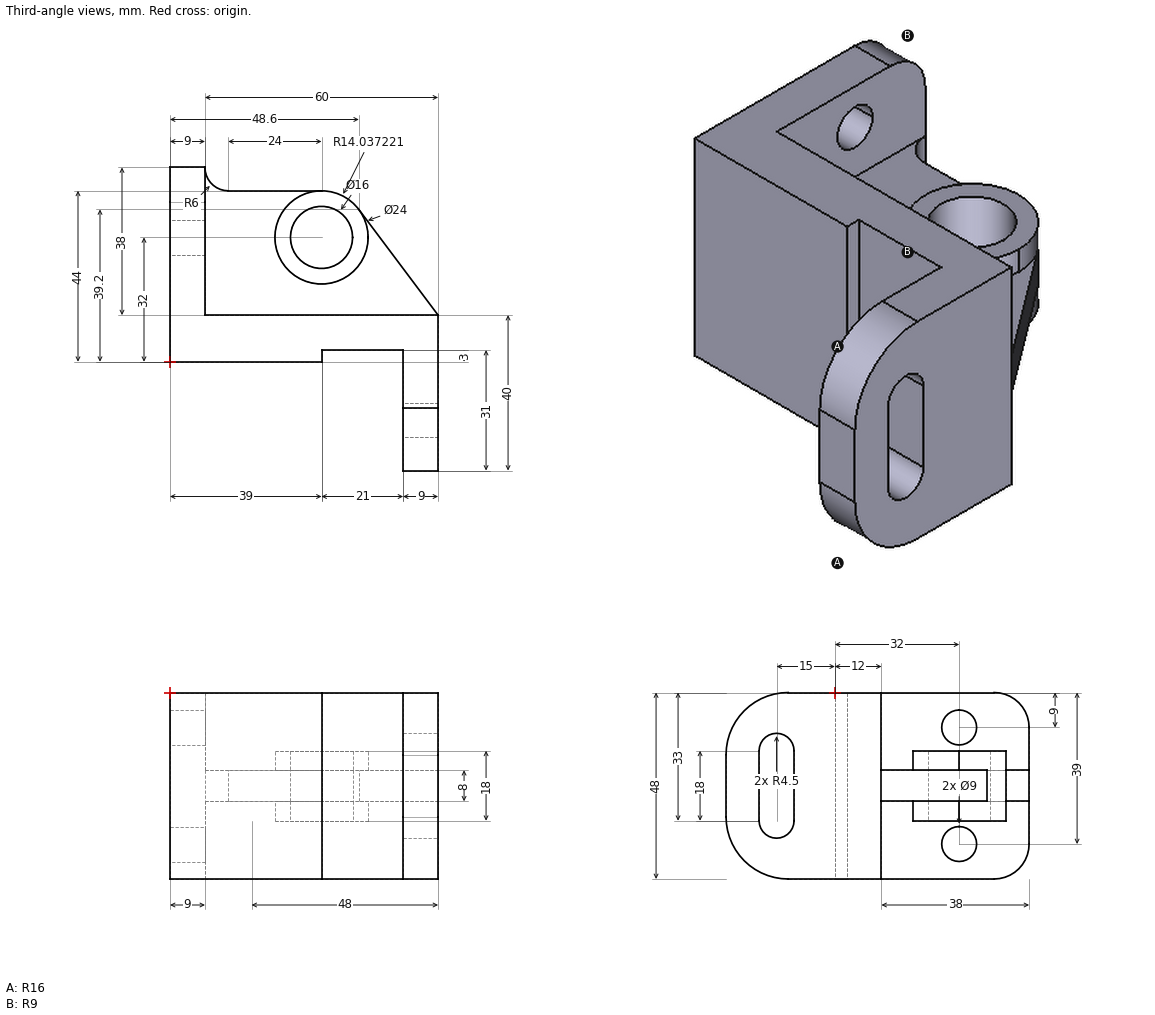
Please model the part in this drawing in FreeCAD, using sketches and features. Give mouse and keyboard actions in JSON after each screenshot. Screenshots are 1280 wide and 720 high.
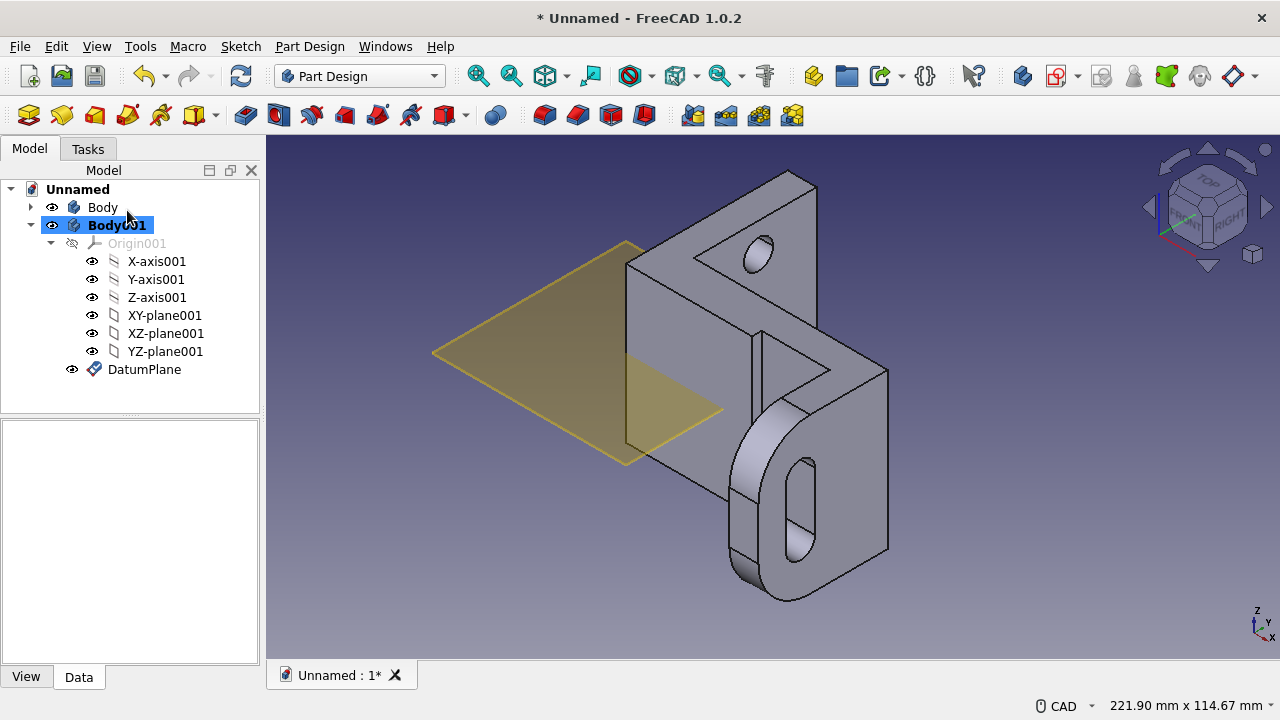
{"action": "left_click", "coordinate": [117, 369]}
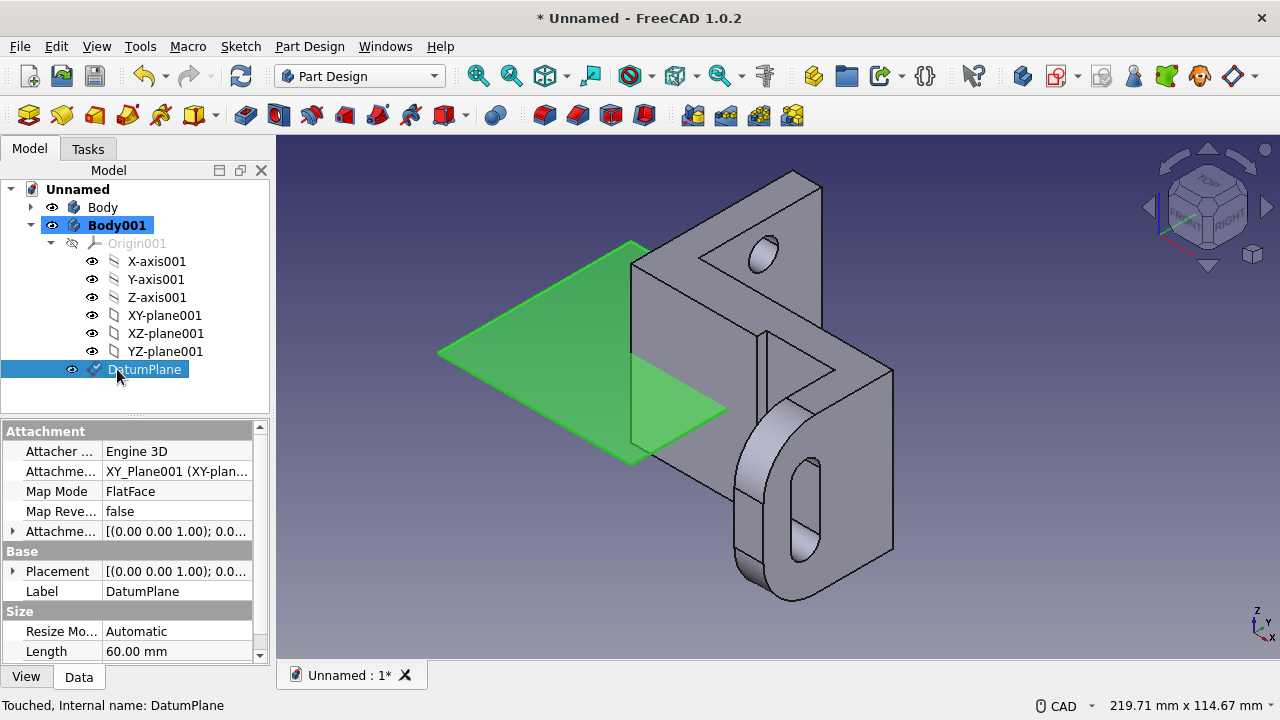
{"action": "left_click", "coordinate": [1056, 76]}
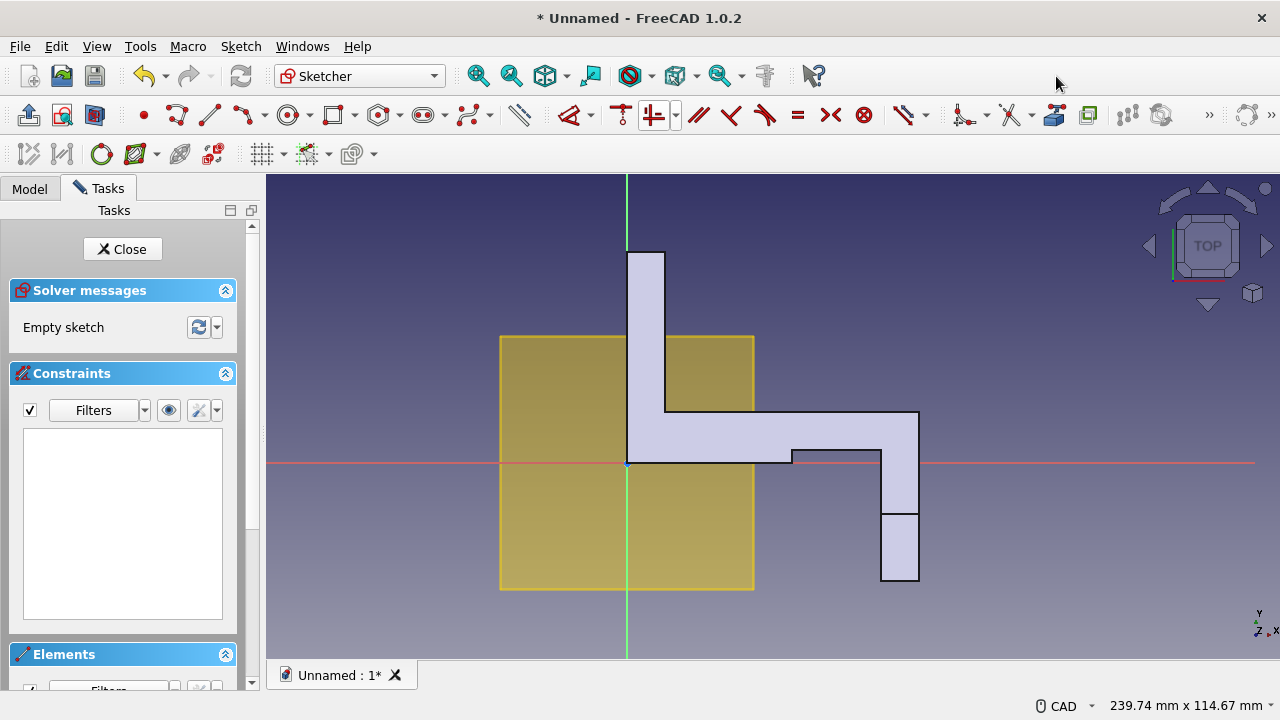
{"action": "scroll", "coordinate": [797, 275], "scroll_direction": "up", "scroll_amount": 2}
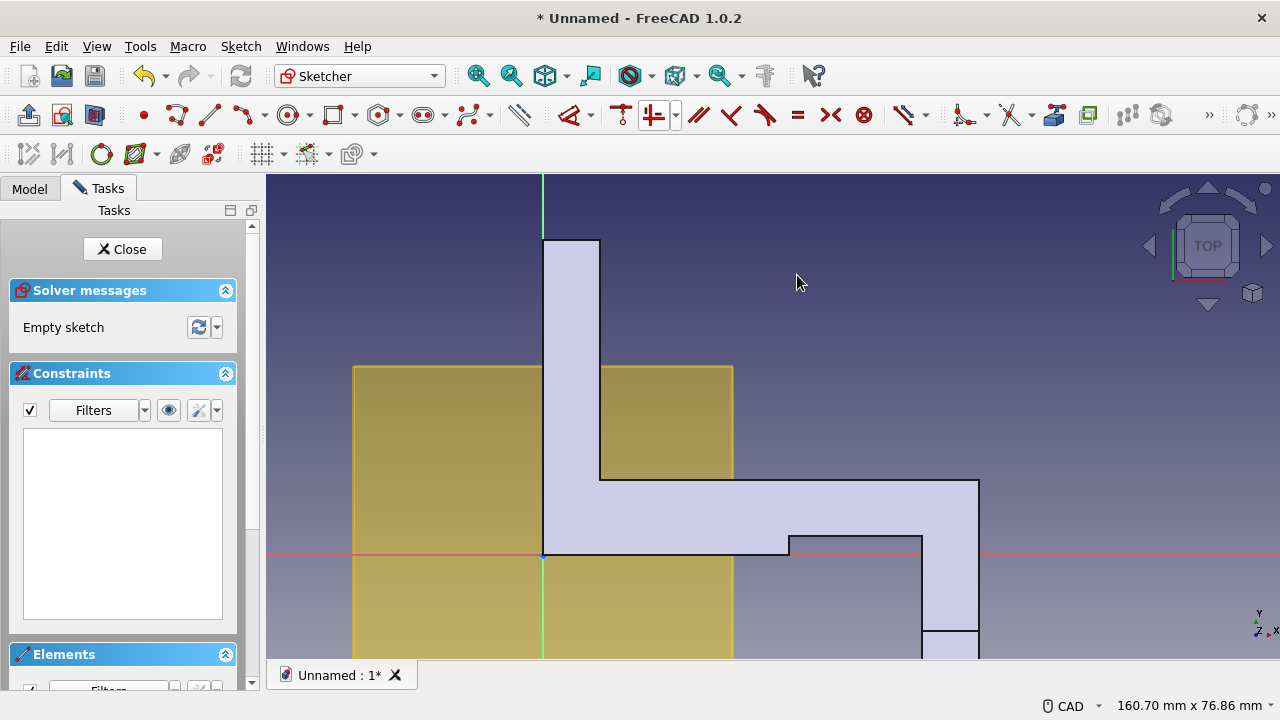
{"action": "key", "text": "g c"}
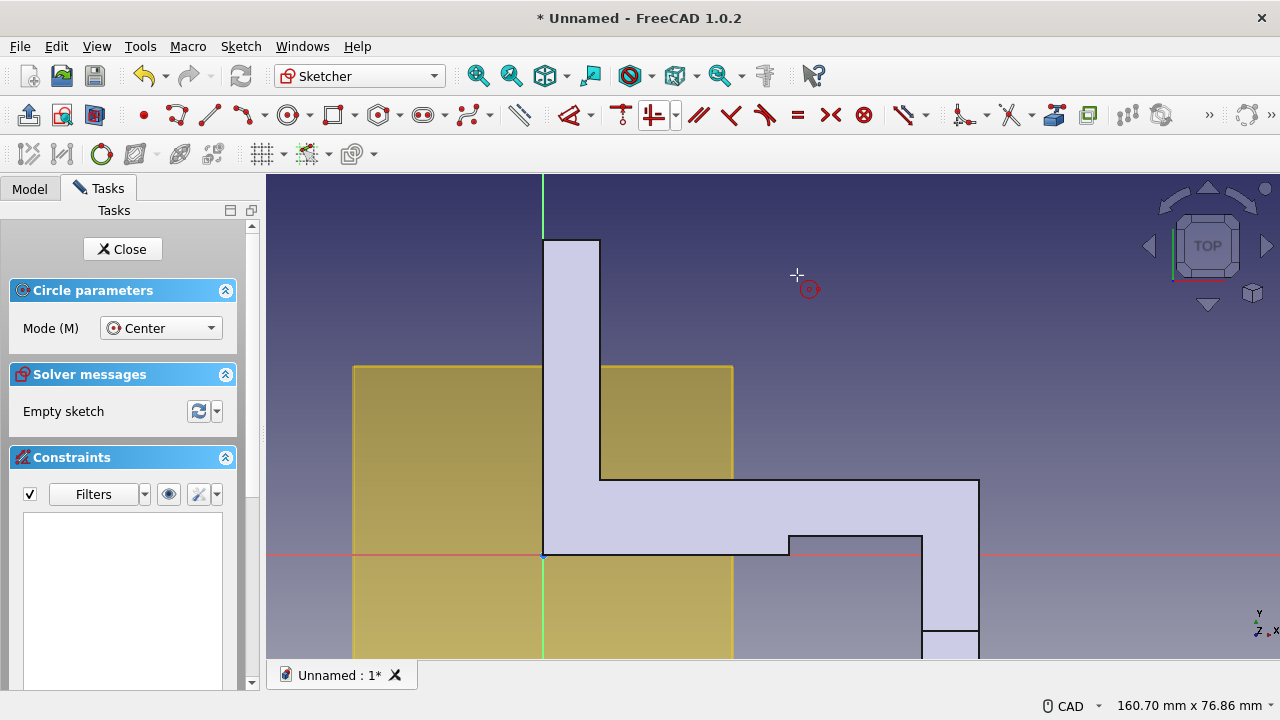
{"action": "left_click", "coordinate": [789, 353]}
{"action": "left_click", "coordinate": [843, 300]}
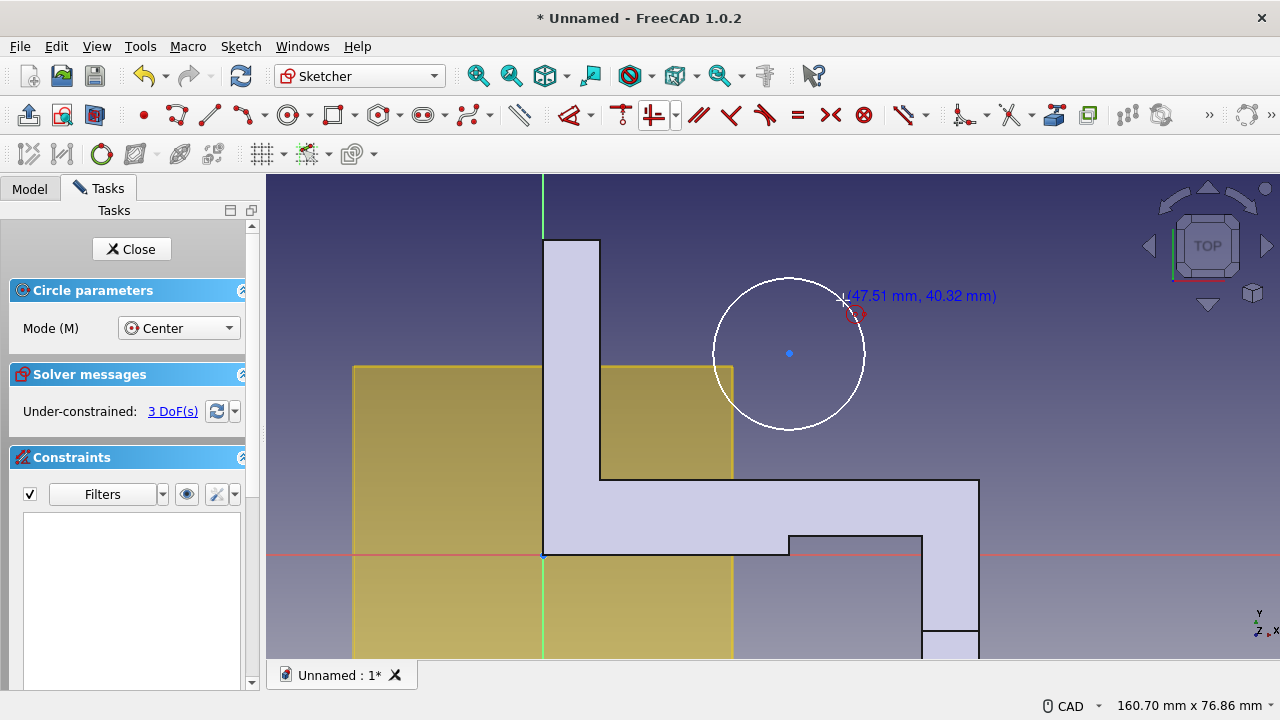
{"action": "left_click", "coordinate": [789, 354]}
{"action": "left_click", "coordinate": [825, 318]}
{"action": "key", "text": "Escape"}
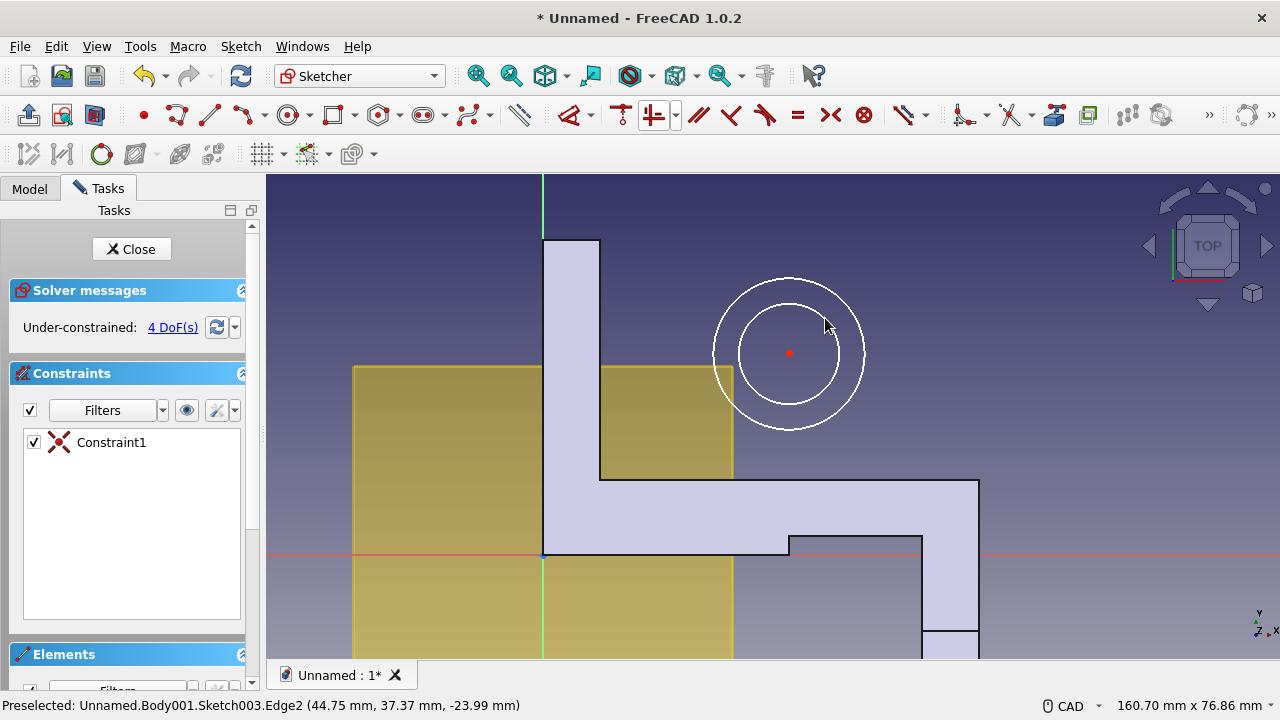
{"action": "key", "text": "d"}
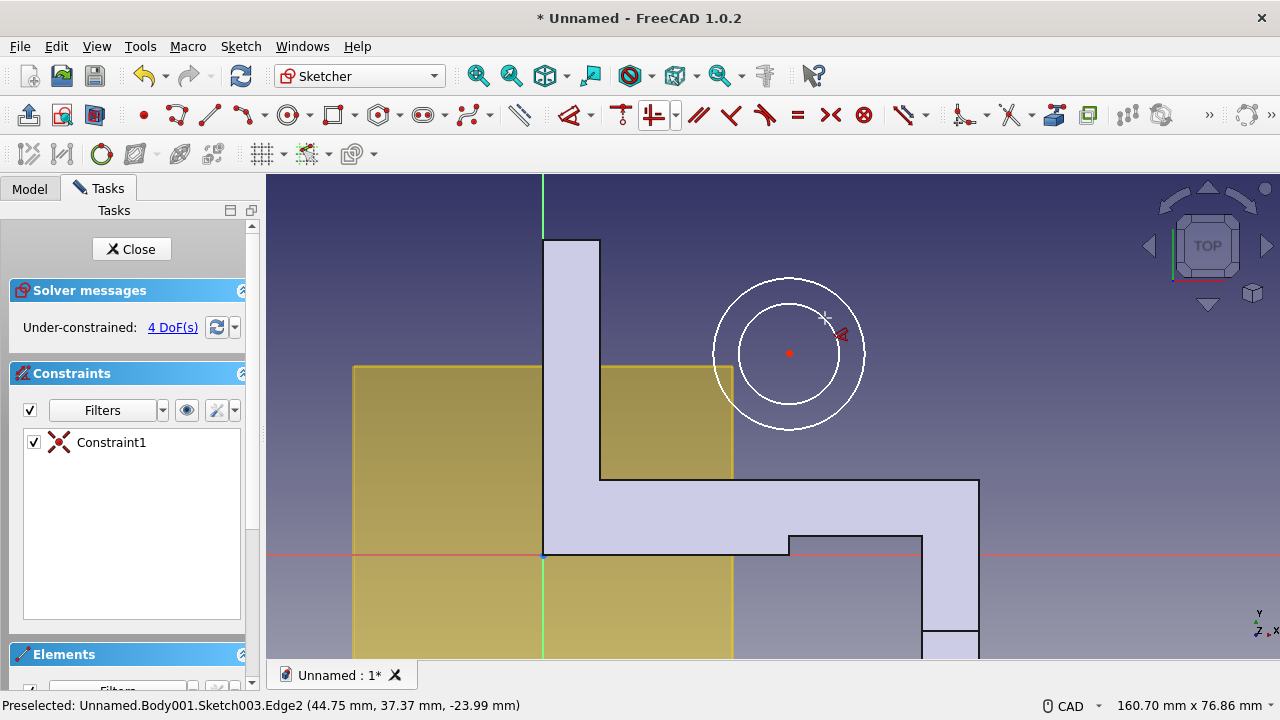
{"action": "left_click", "coordinate": [842, 300]}
{"action": "left_click", "coordinate": [864, 277]}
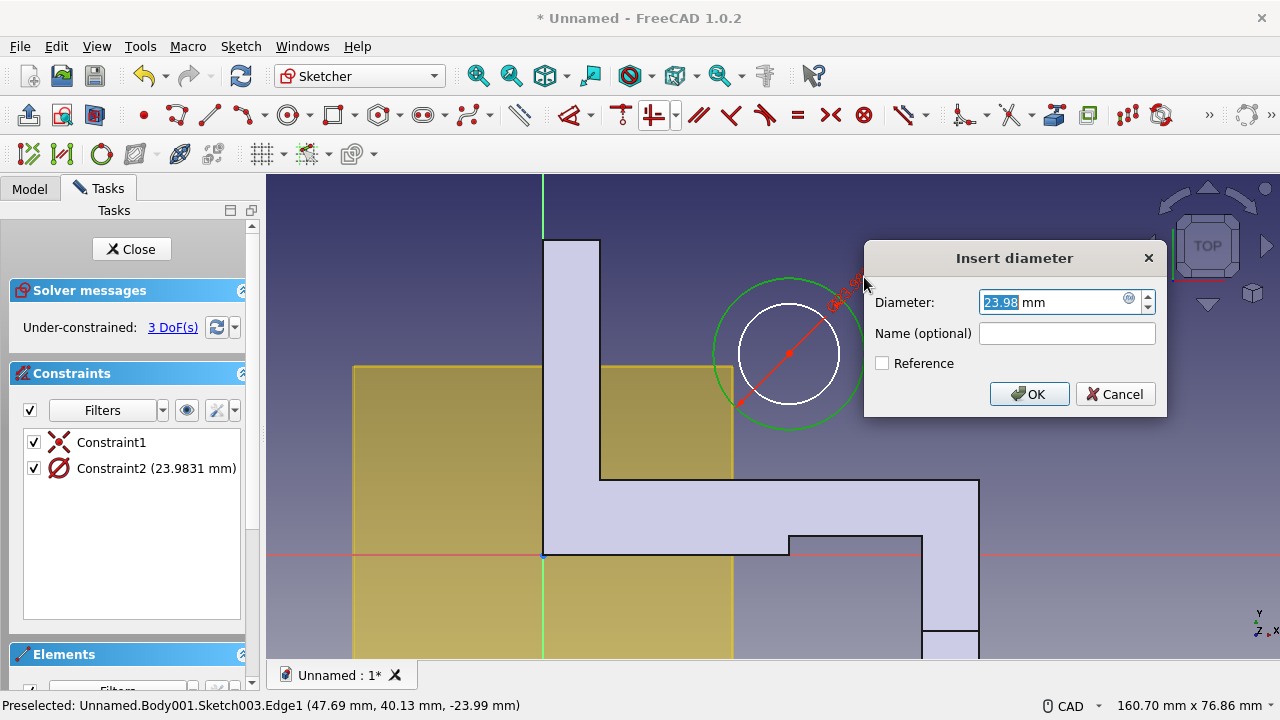
{"action": "type", "text": "24"}
{"action": "key", "text": "Return"}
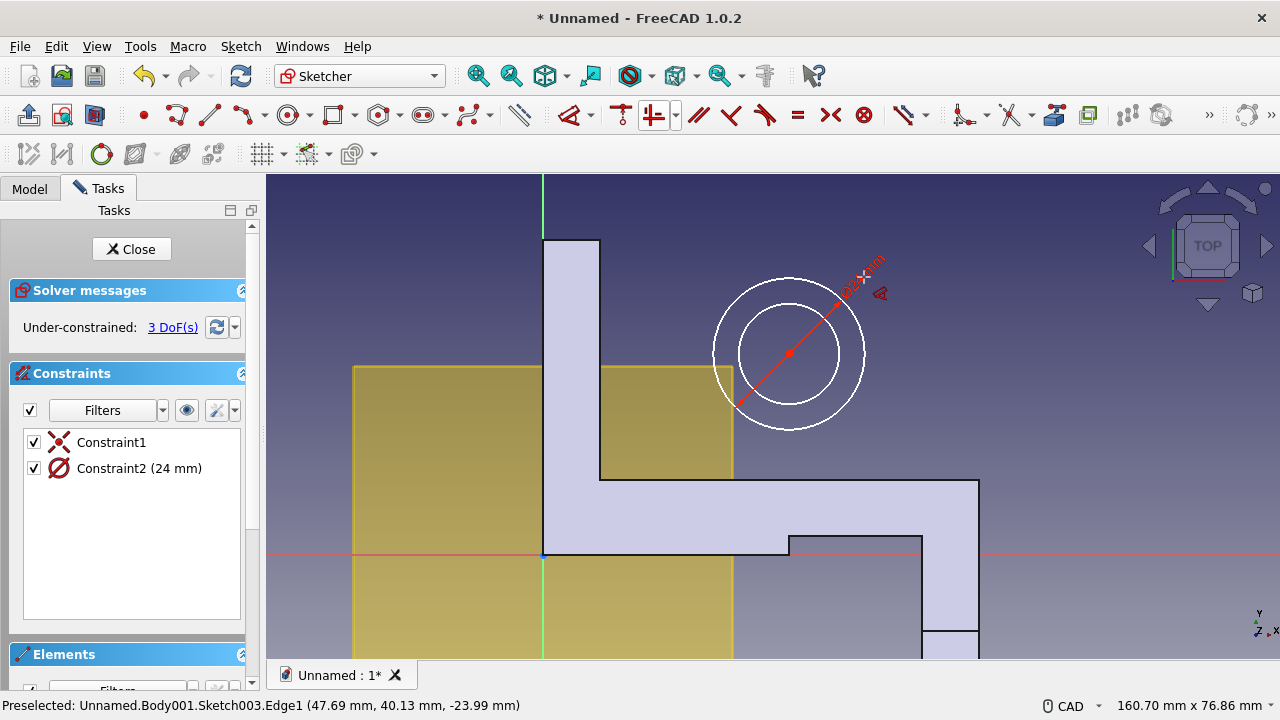
{"action": "left_click", "coordinate": [824, 318]}
{"action": "left_click", "coordinate": [890, 323]}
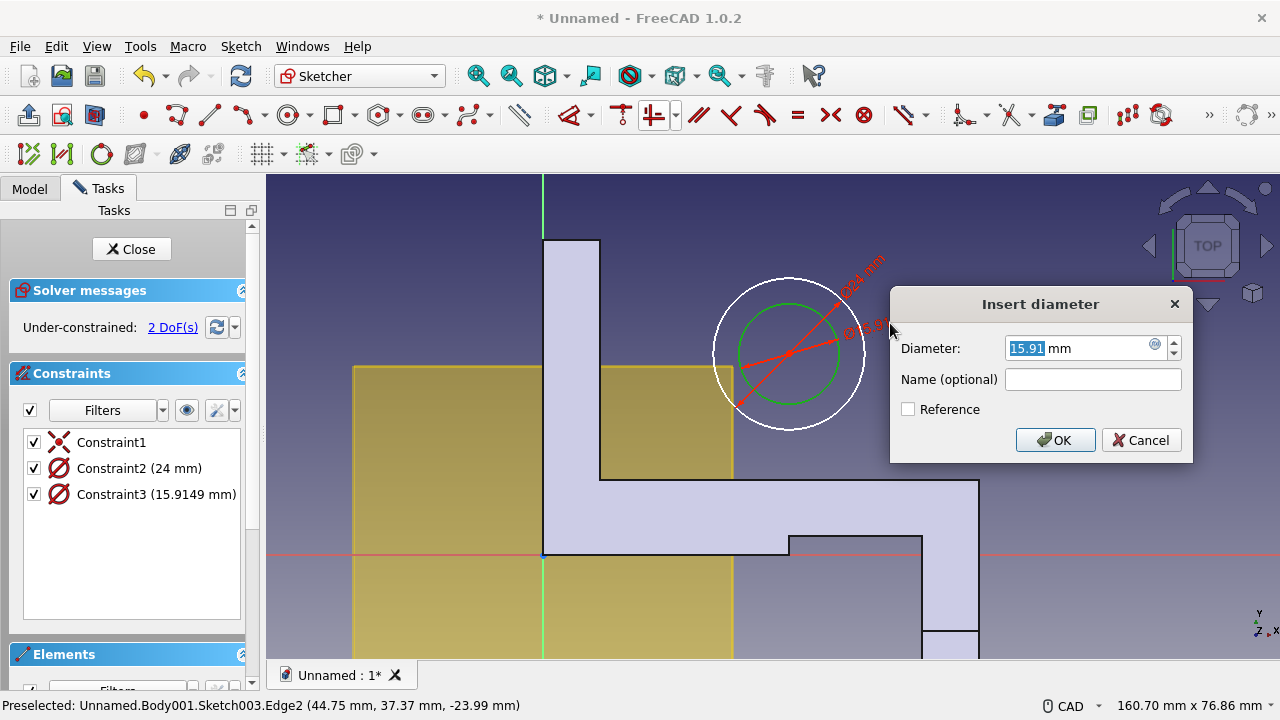
{"action": "type", "text": "16"}
{"action": "key", "text": "Return"}